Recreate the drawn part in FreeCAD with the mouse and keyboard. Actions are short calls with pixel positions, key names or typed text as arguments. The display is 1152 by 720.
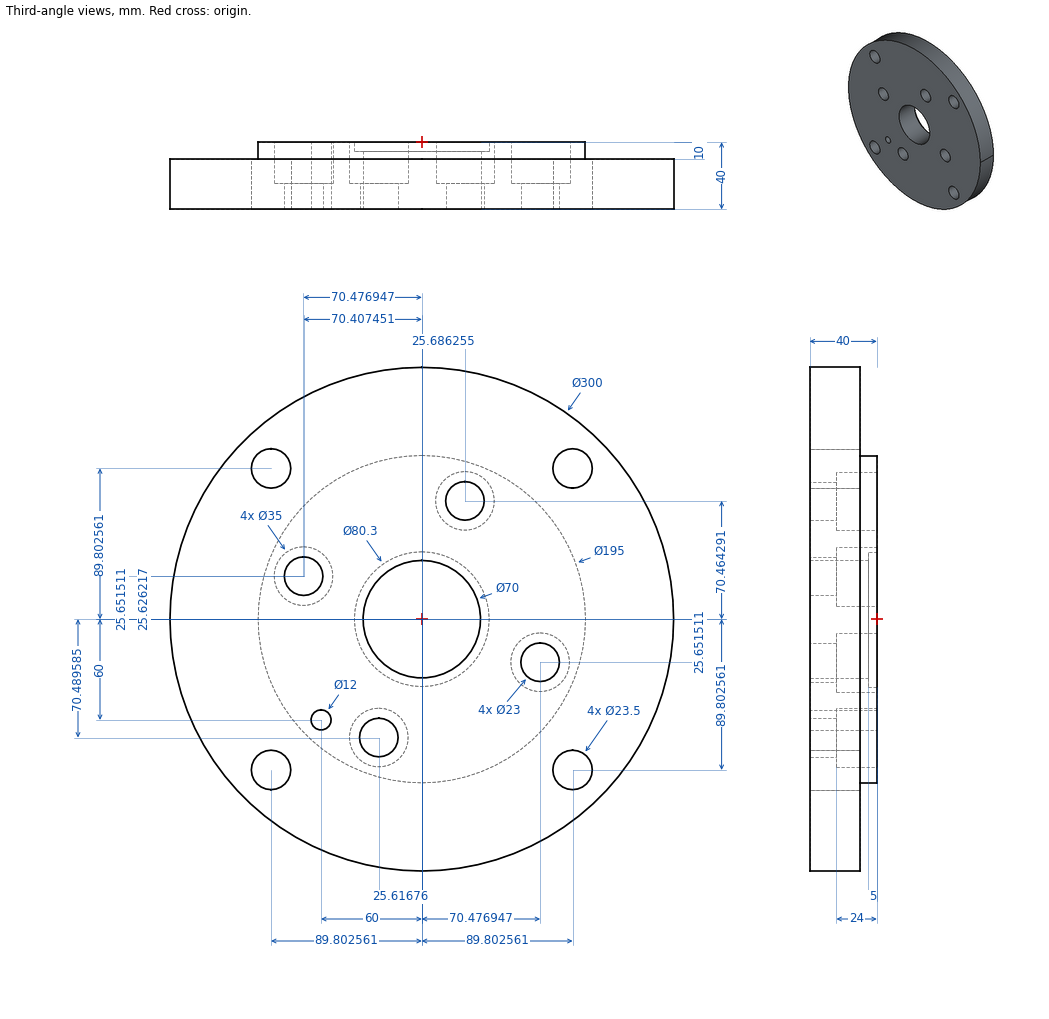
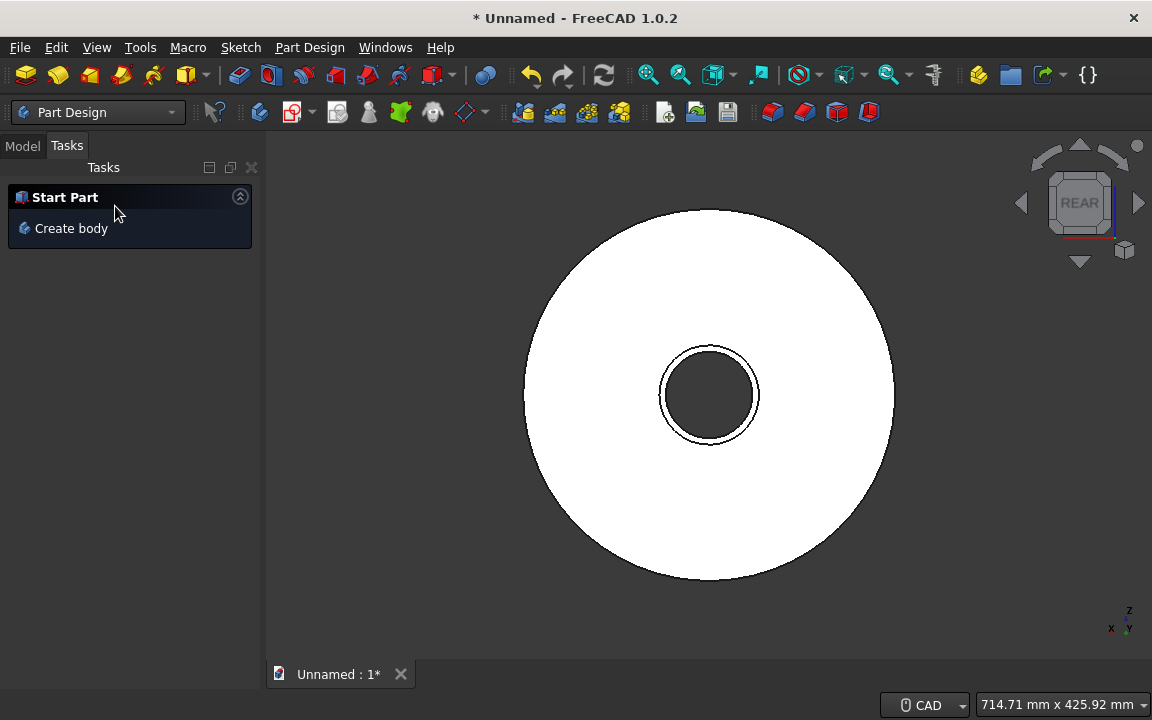
click(292, 112)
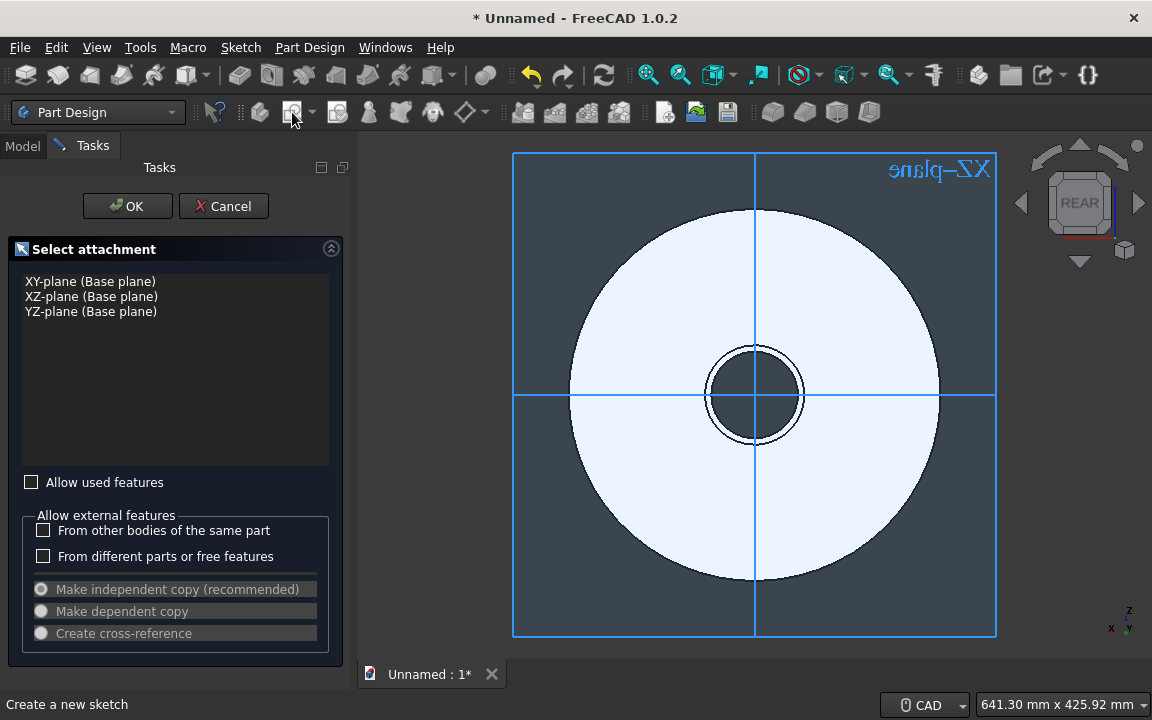
click(82, 296)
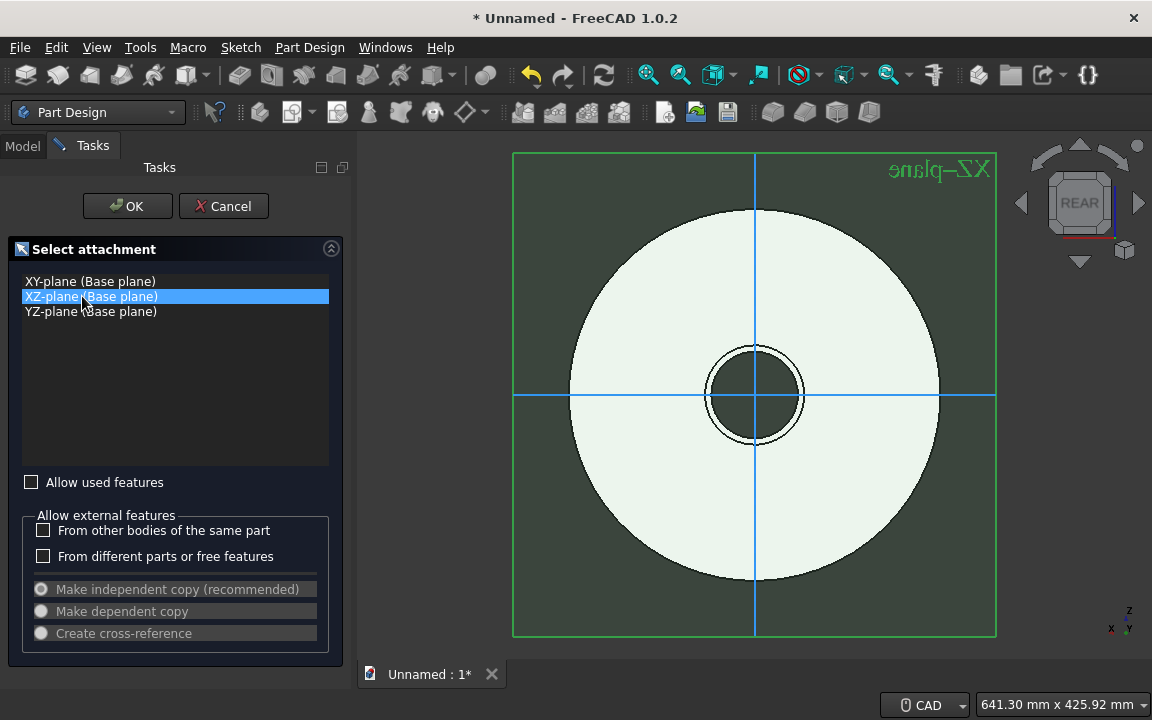
click(128, 206)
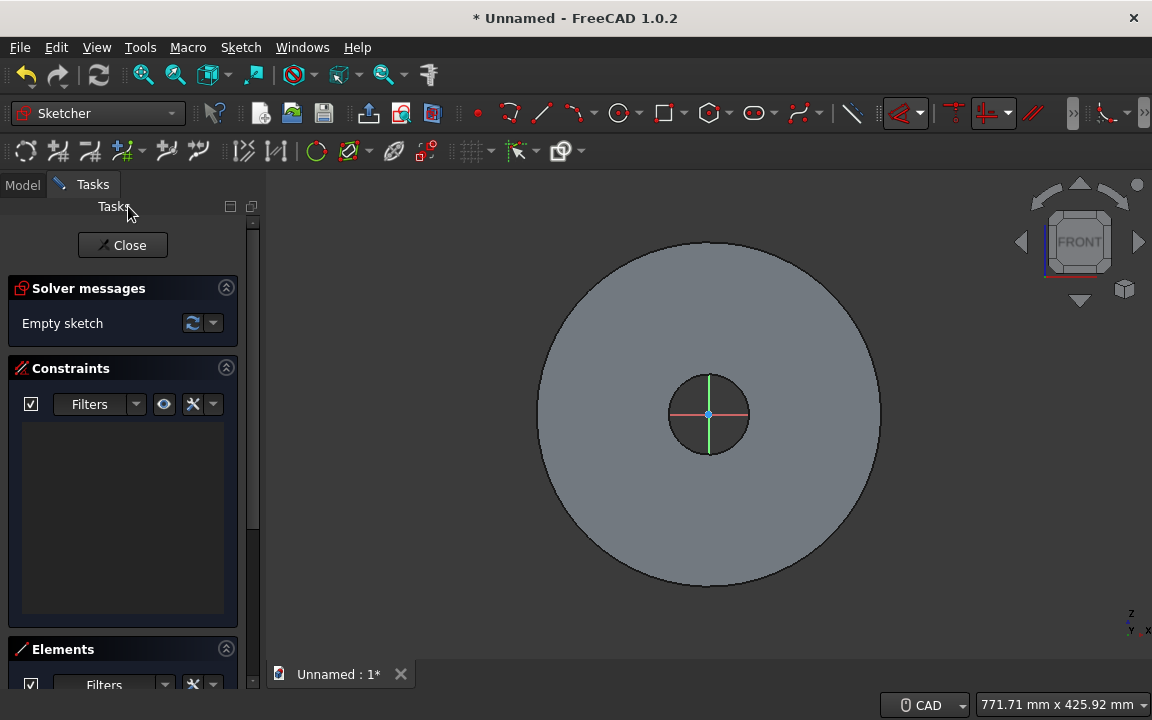
click(434, 114)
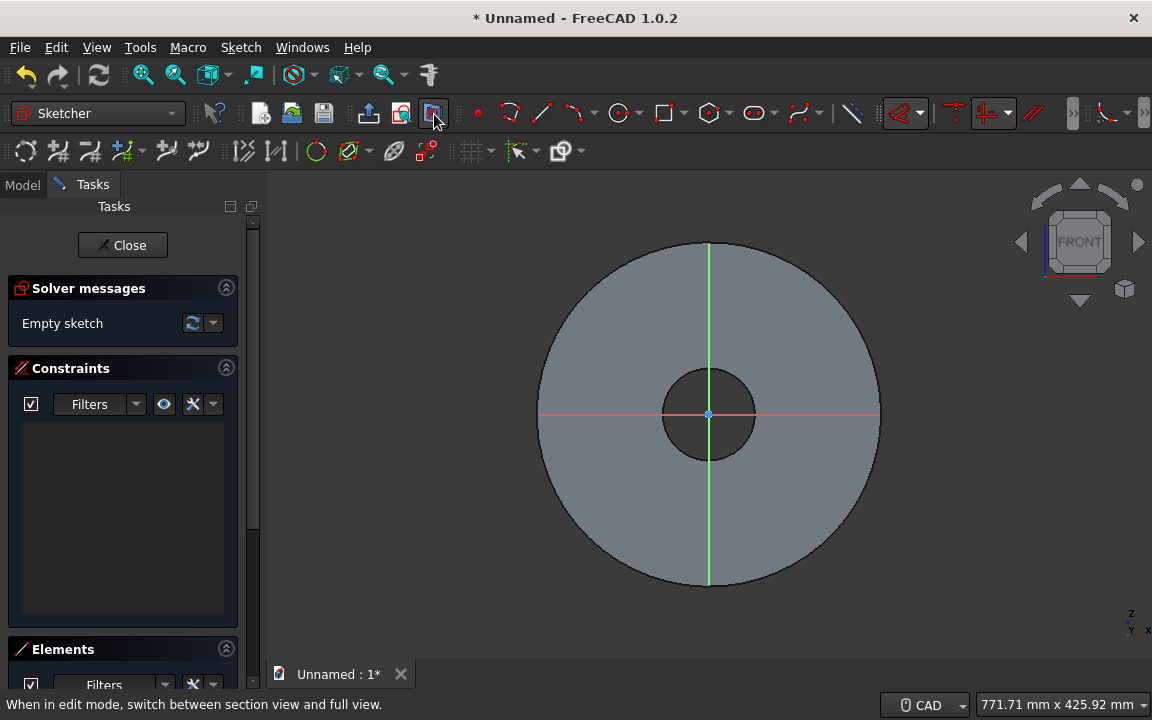
click(620, 114)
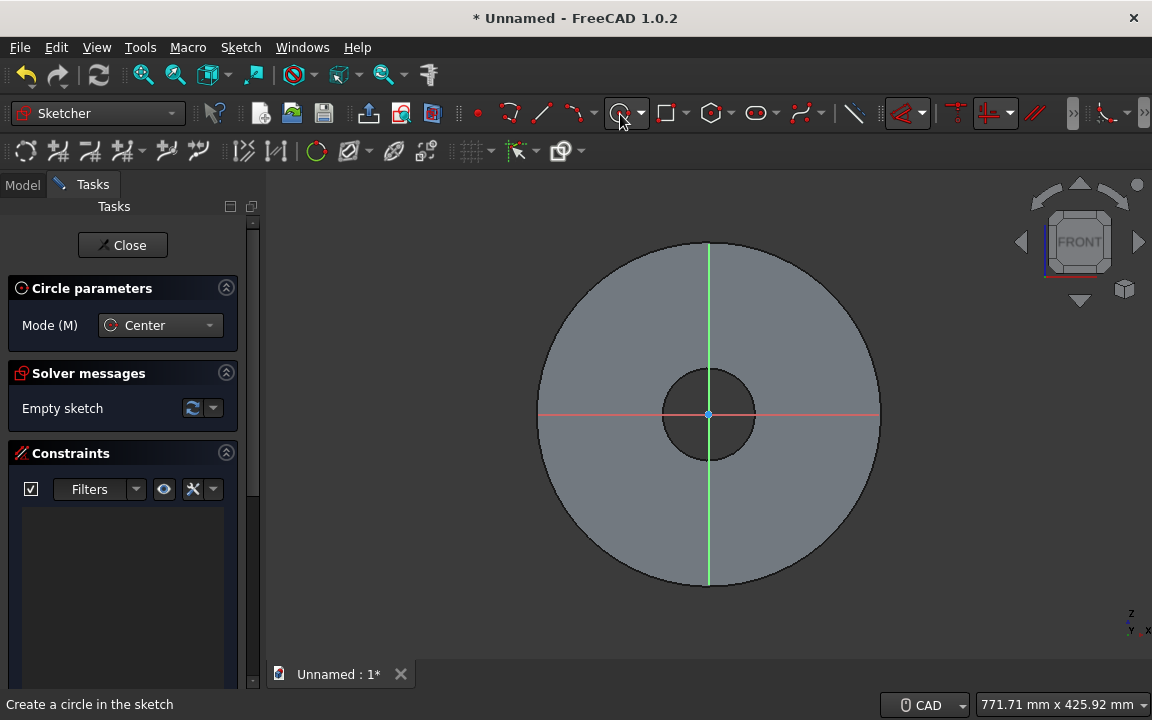
click(709, 415)
move(831, 293)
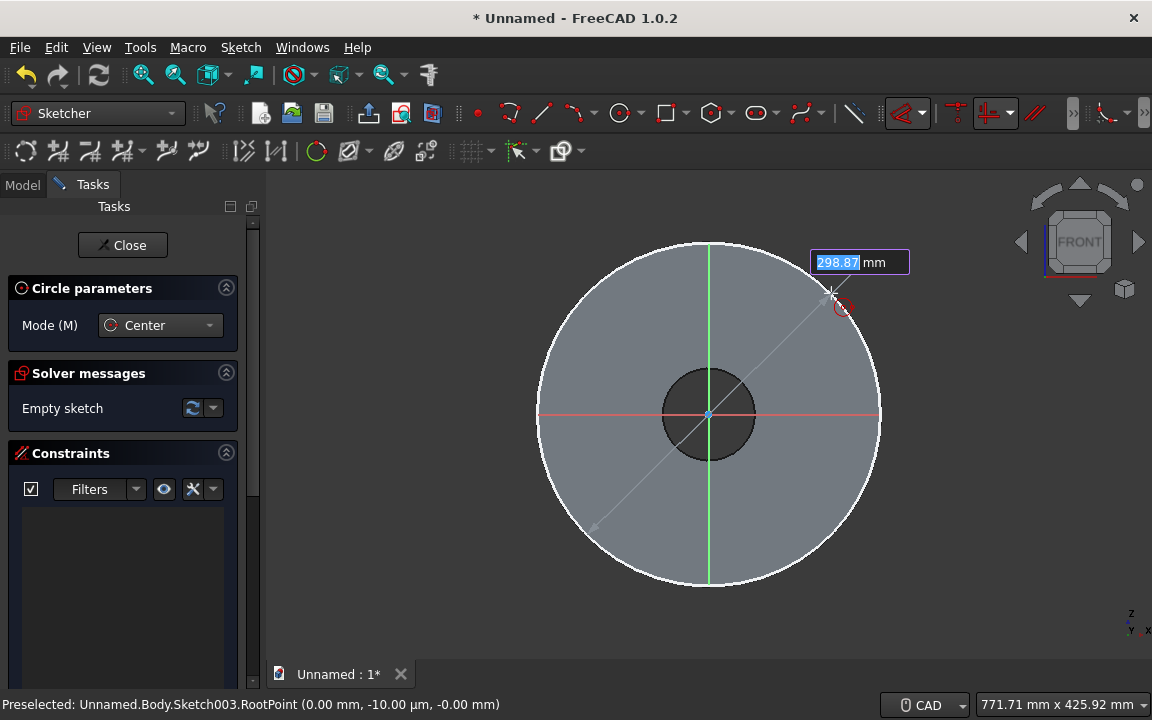
text(300)
key(Return)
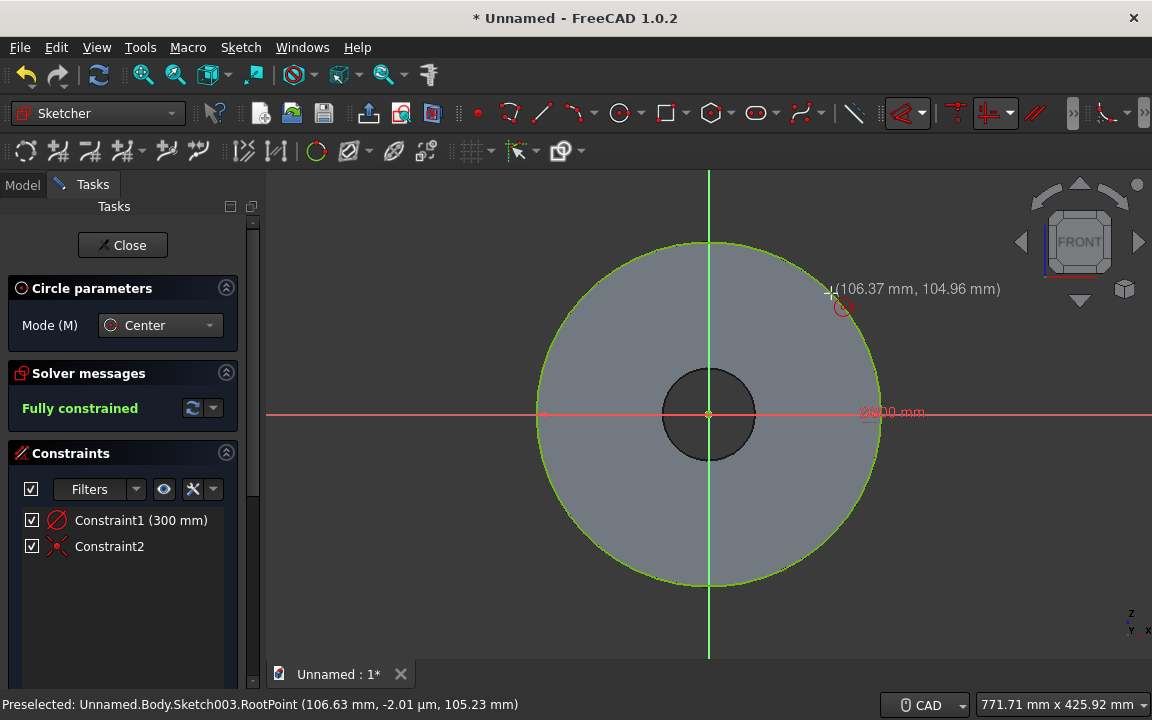
click(709, 415)
move(788, 335)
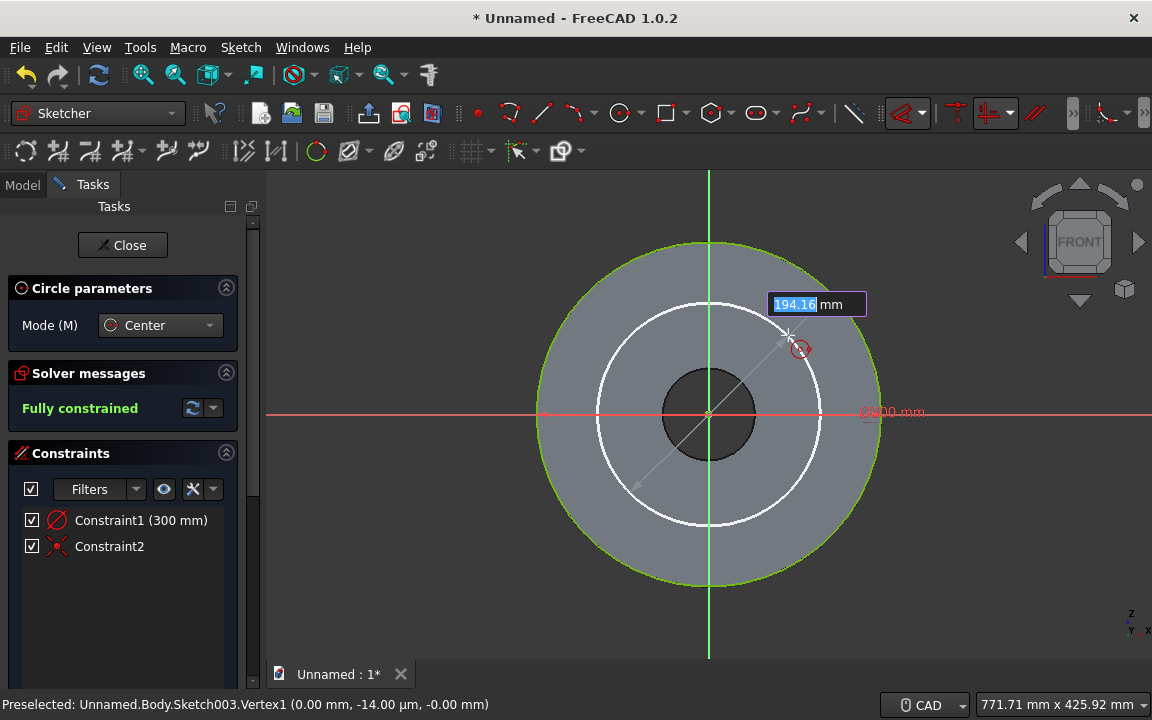
text(195)
key(Return)
key(Escape)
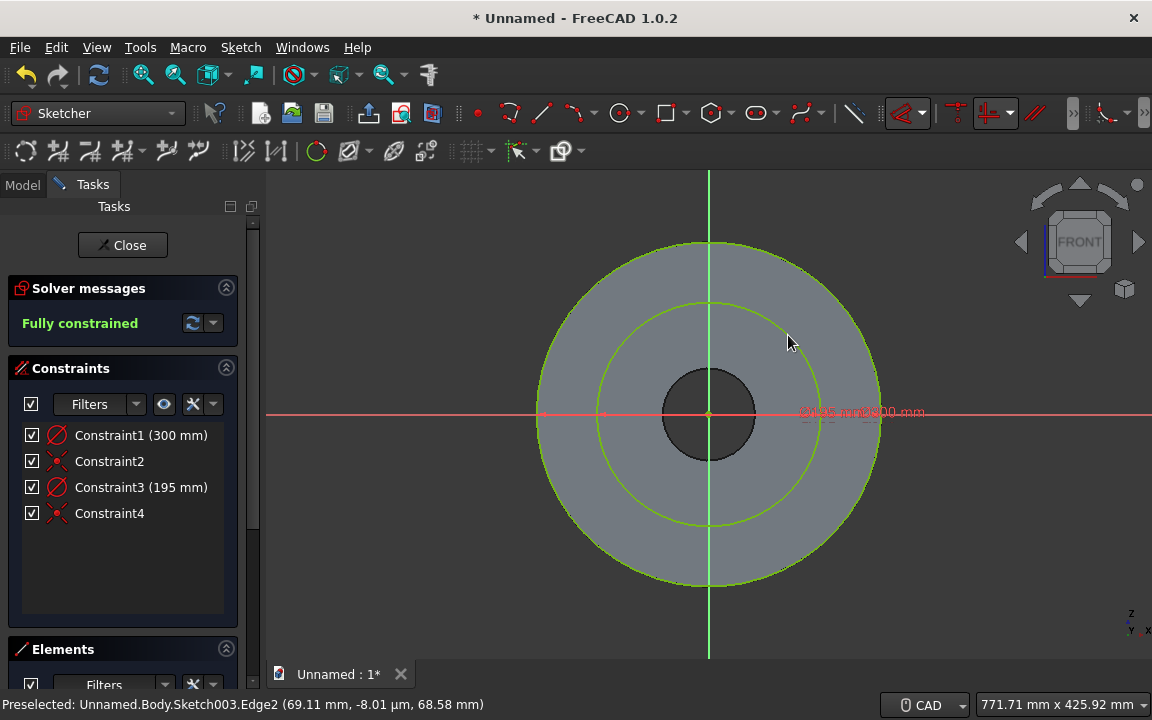
click(123, 245)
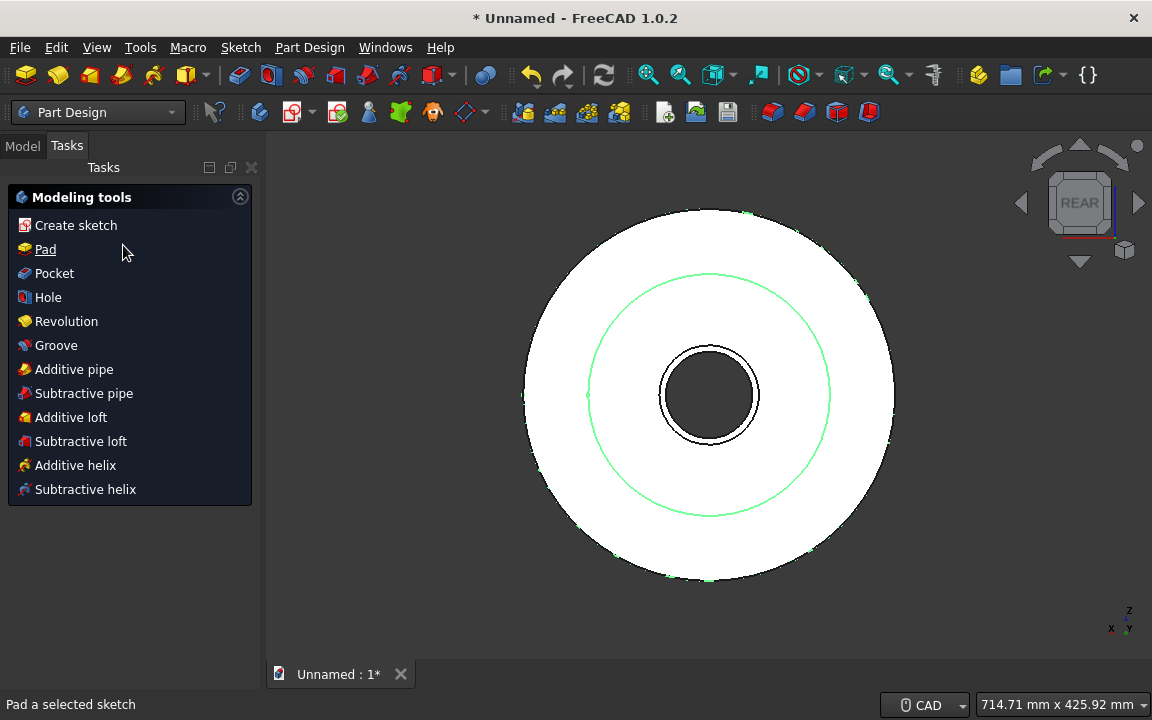
click(240, 76)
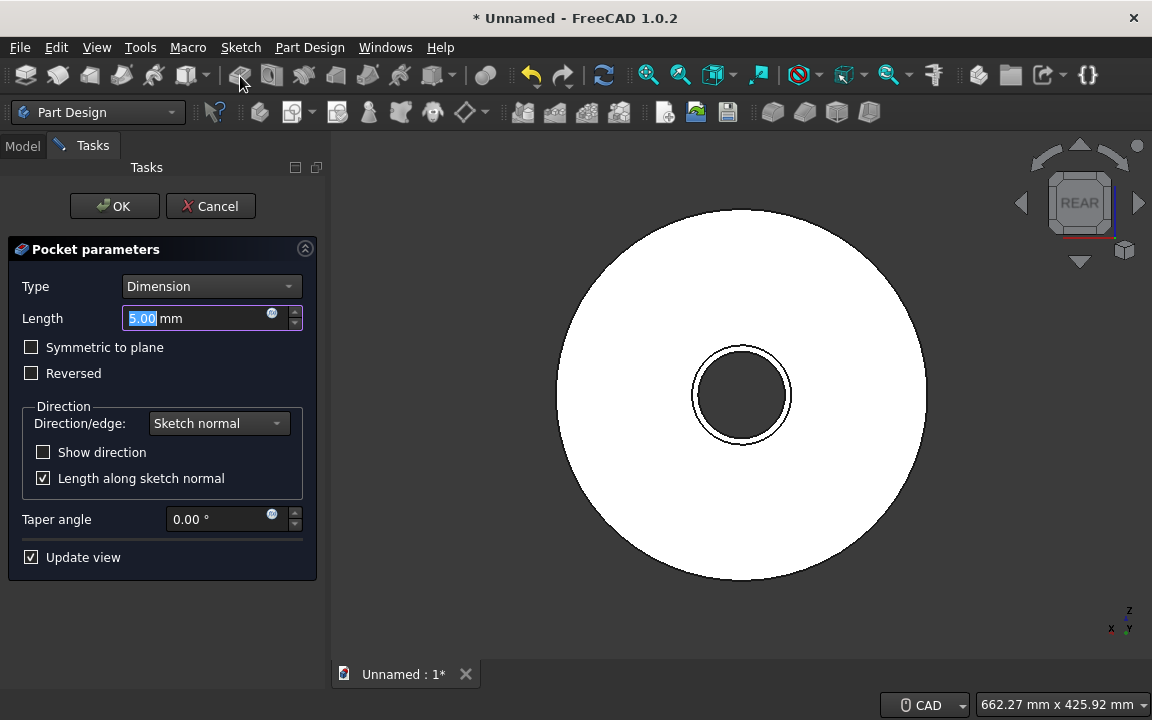
text(10)
key(Tab)